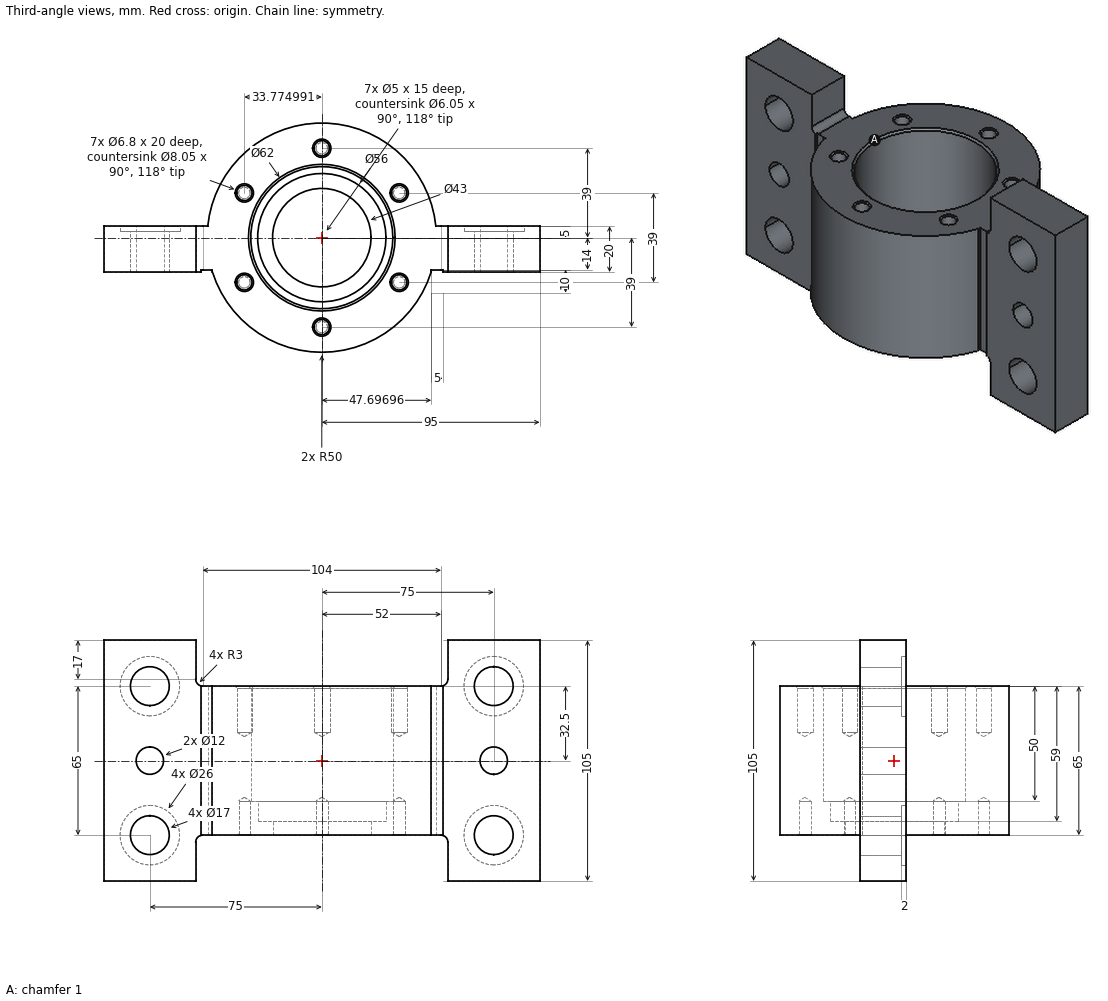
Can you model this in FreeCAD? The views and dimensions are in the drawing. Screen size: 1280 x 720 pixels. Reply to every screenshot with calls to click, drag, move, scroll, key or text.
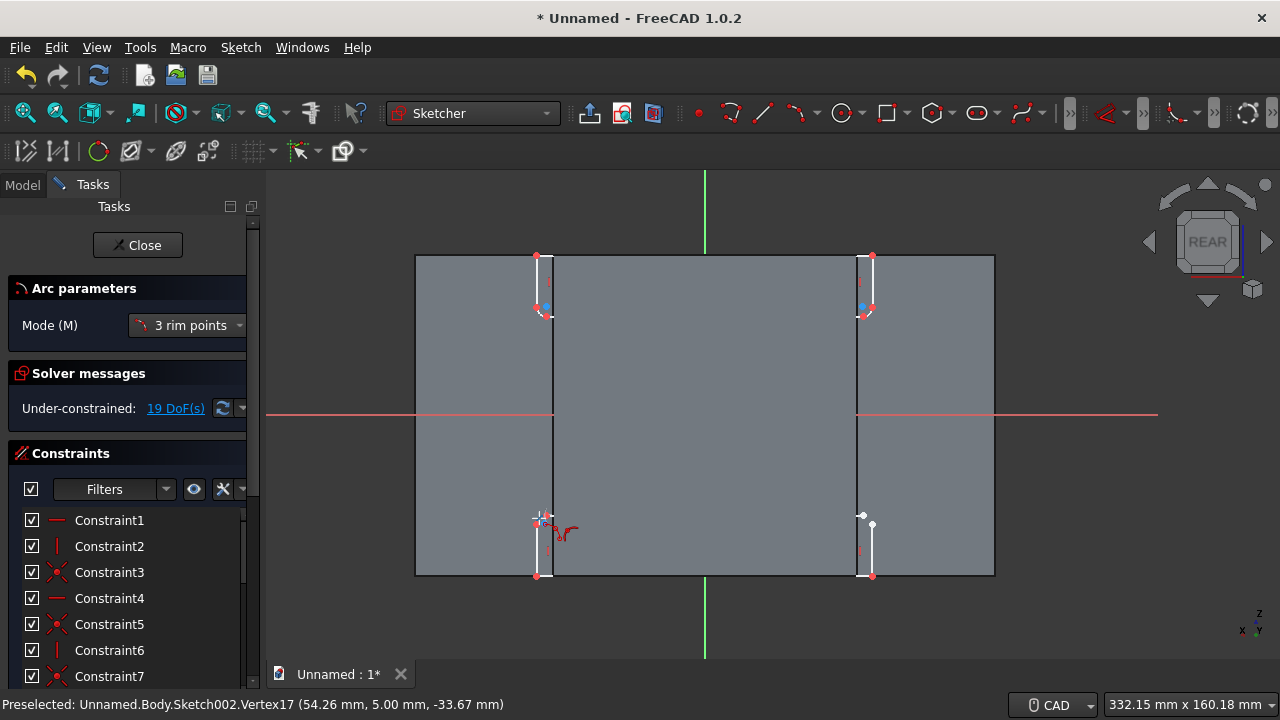
scroll(873, 524, up, 2)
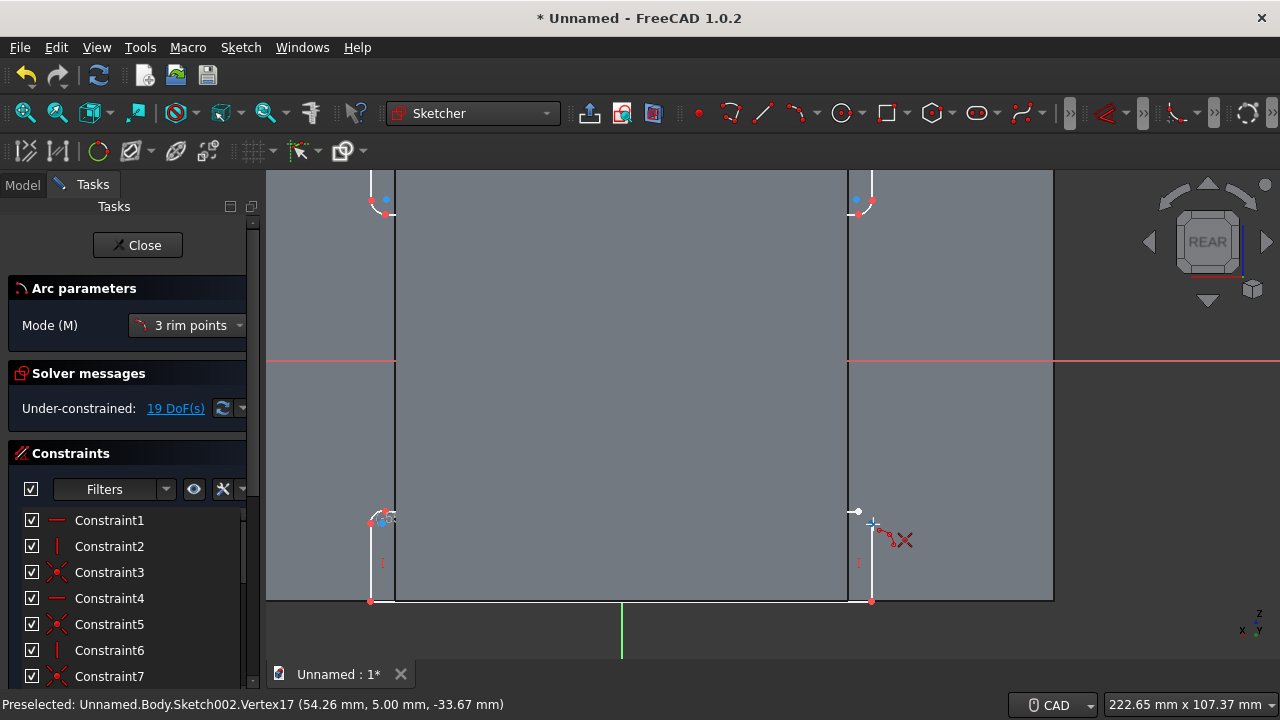
click(872, 524)
click(859, 512)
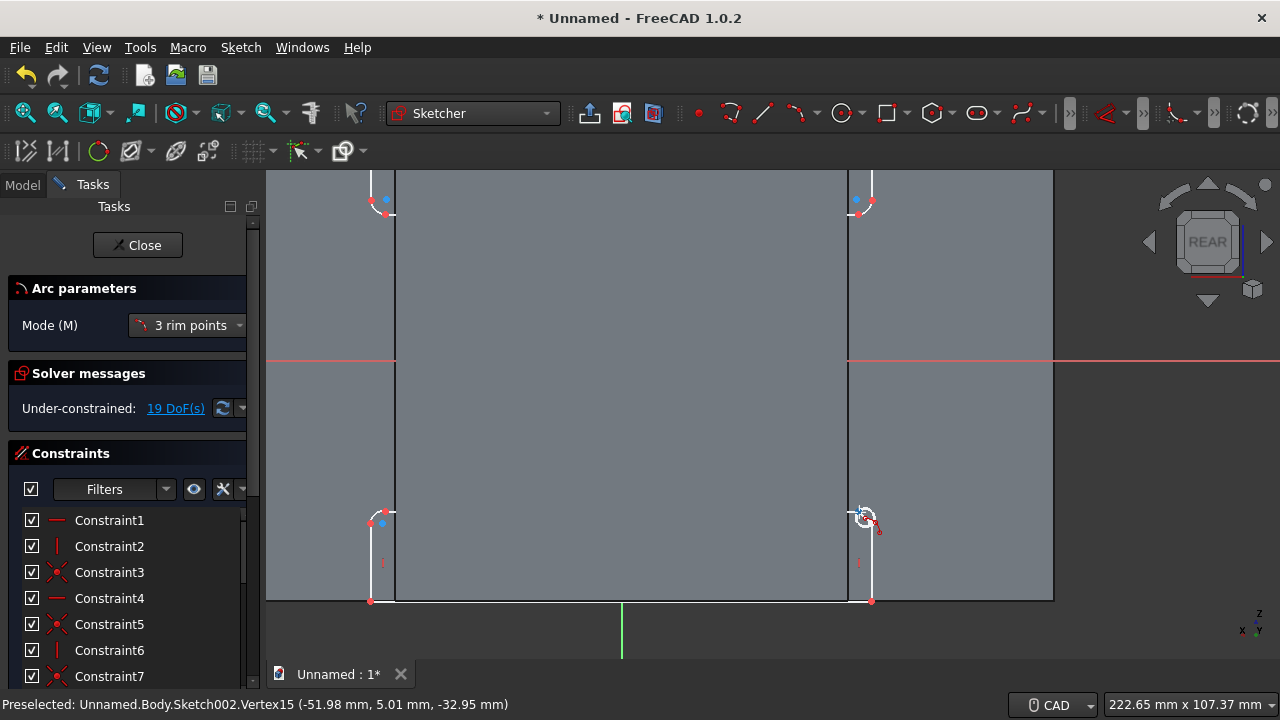
scroll(868, 513, up, 7)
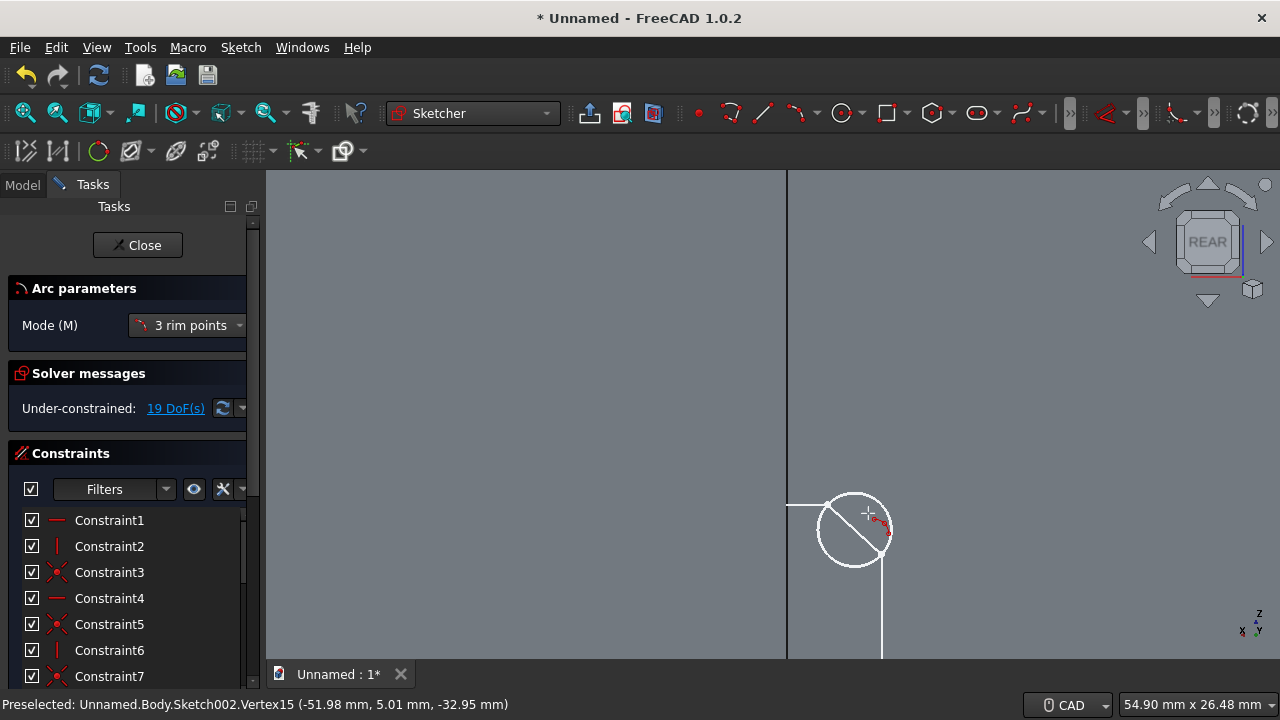
click(867, 513)
key(Escape)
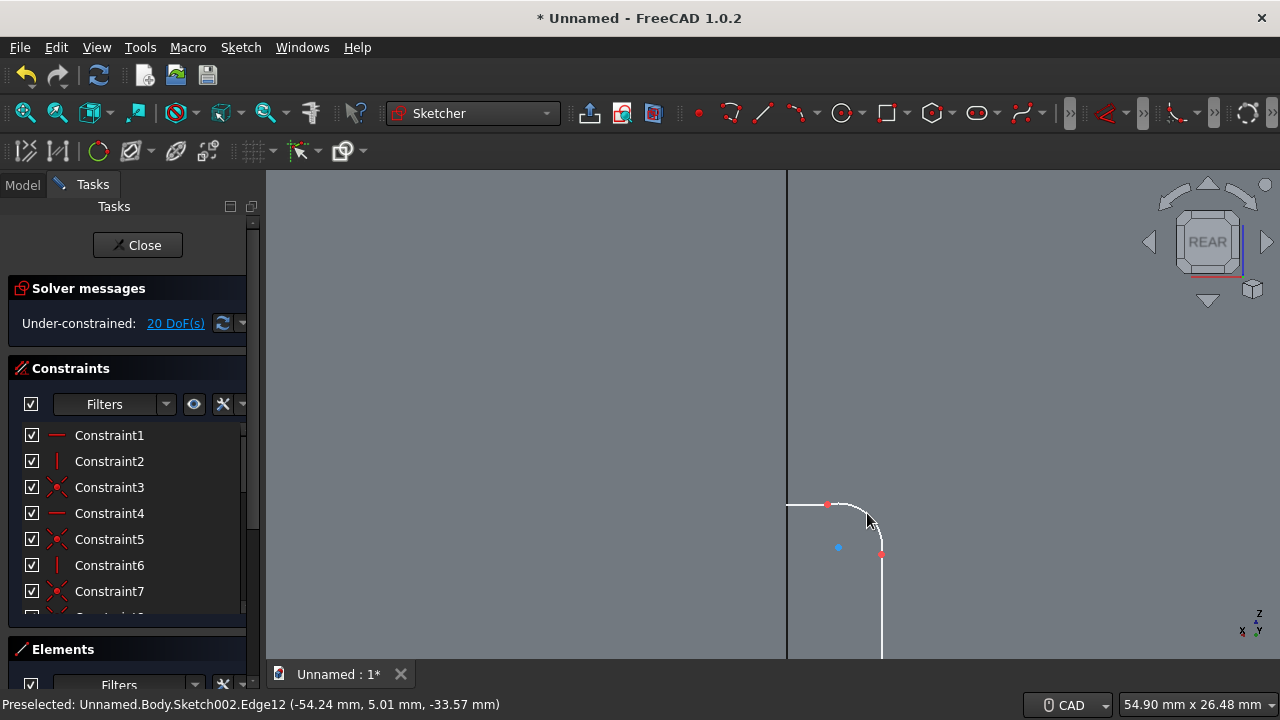
scroll(870, 517, down, 9)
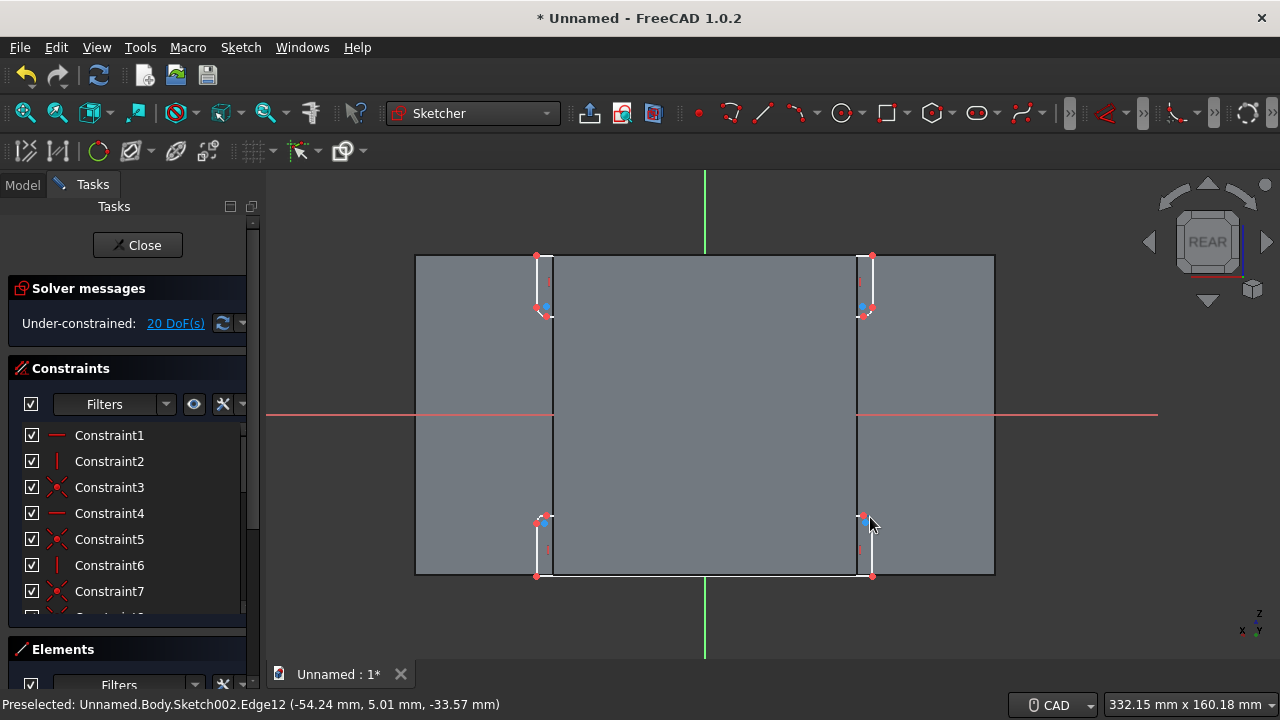
click(642, 317)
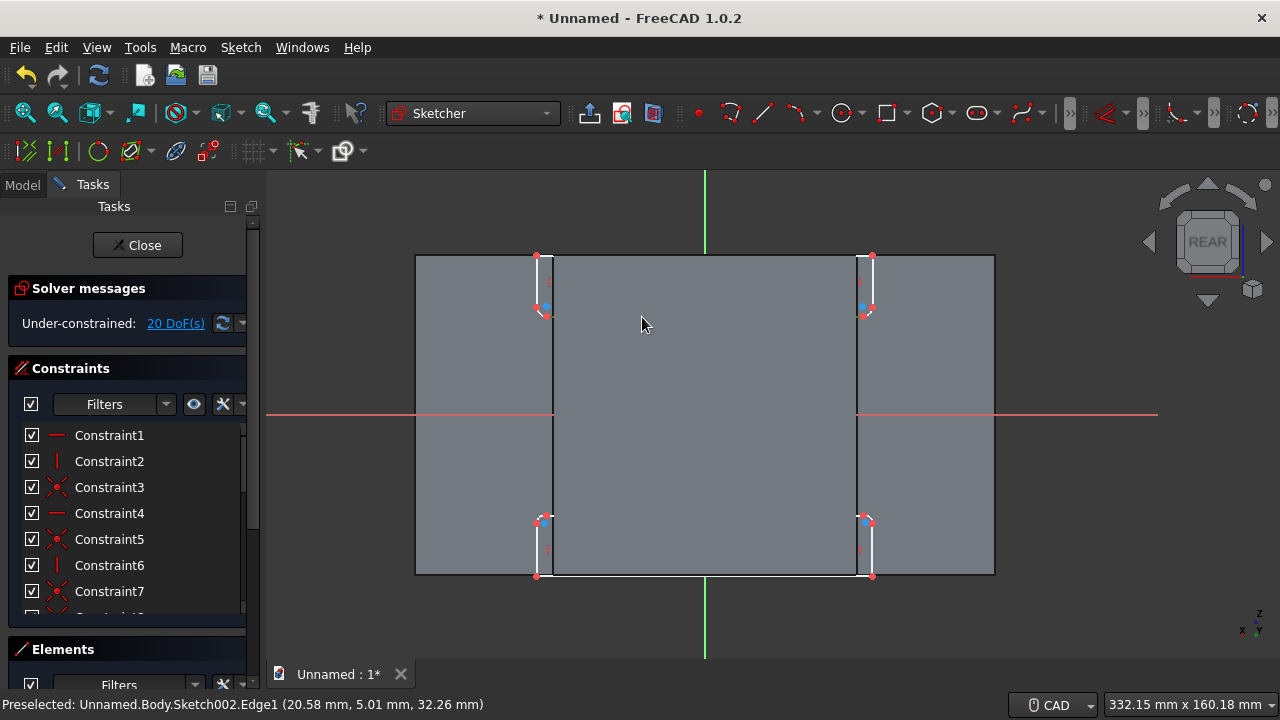
scroll(870, 314, up, 4)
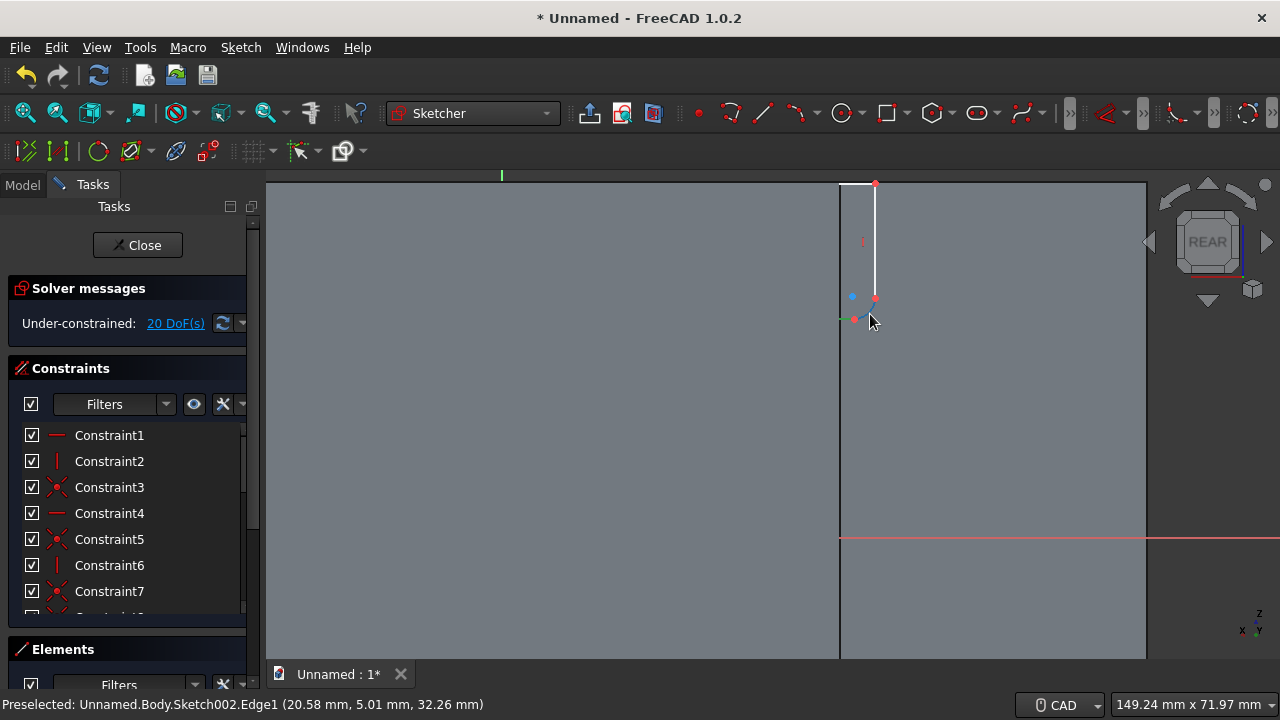
click(869, 313)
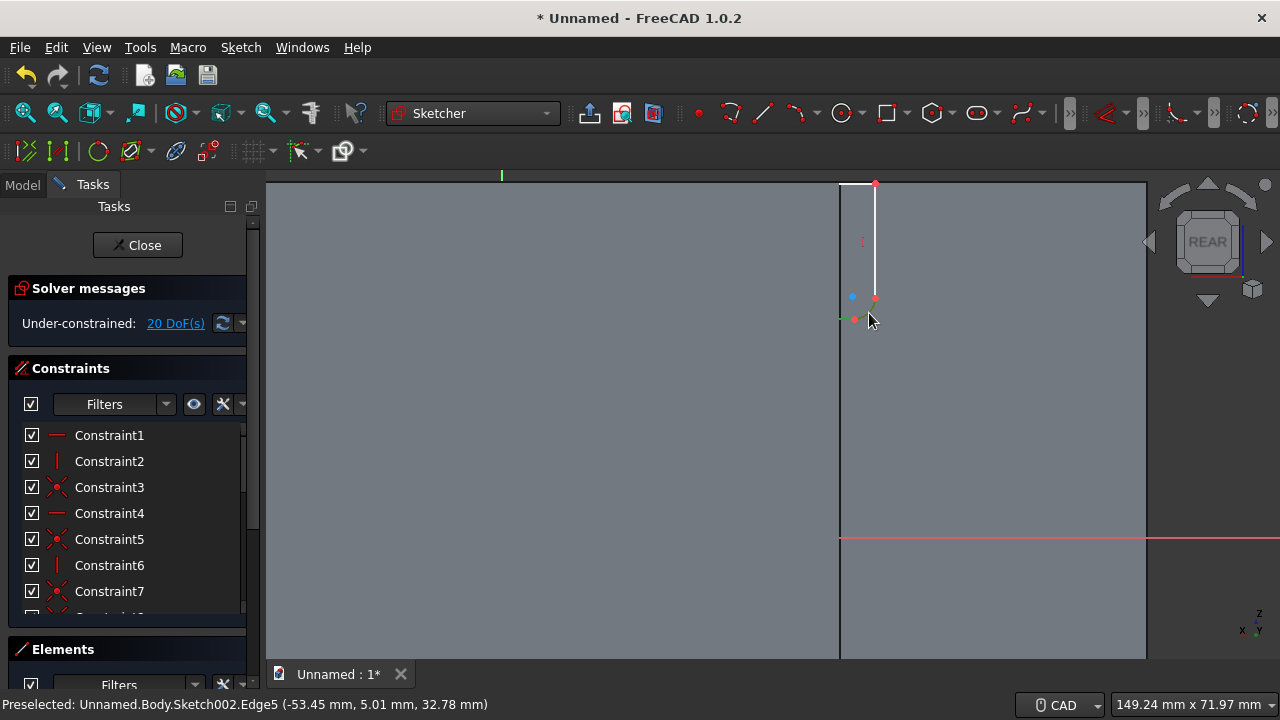
key(t)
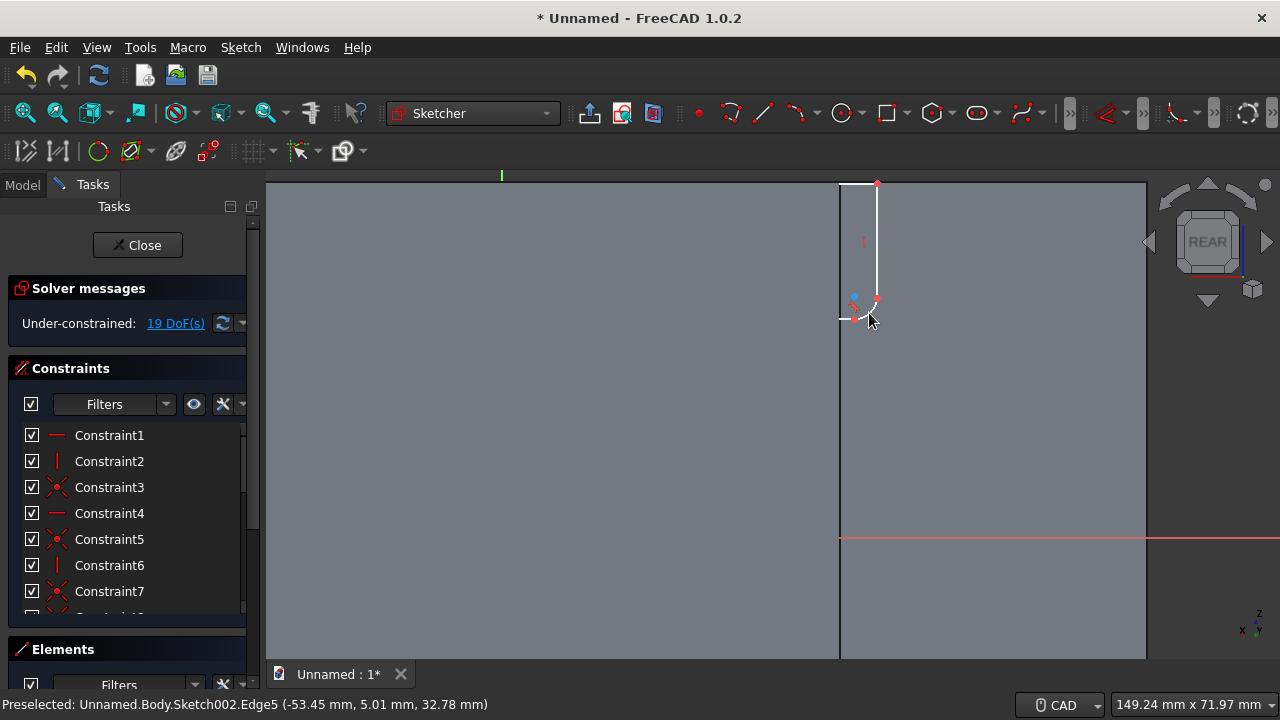
click(361, 319)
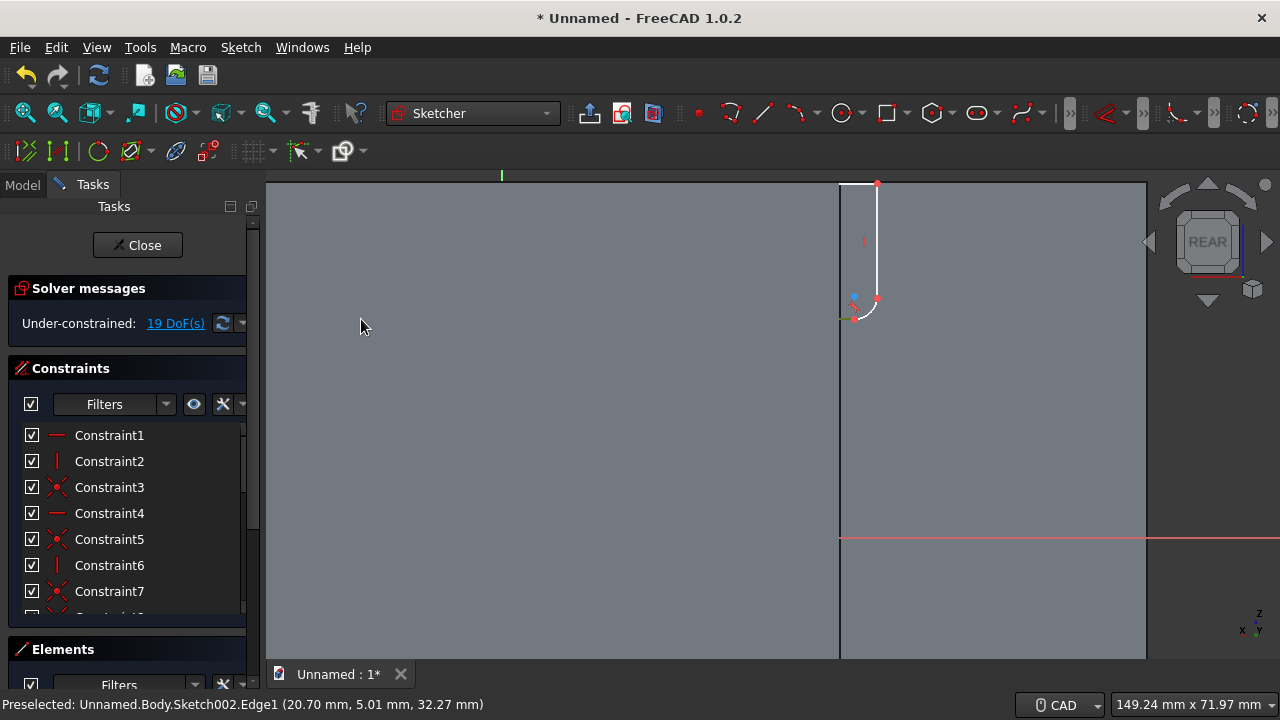
scroll(870, 313, down, 4)